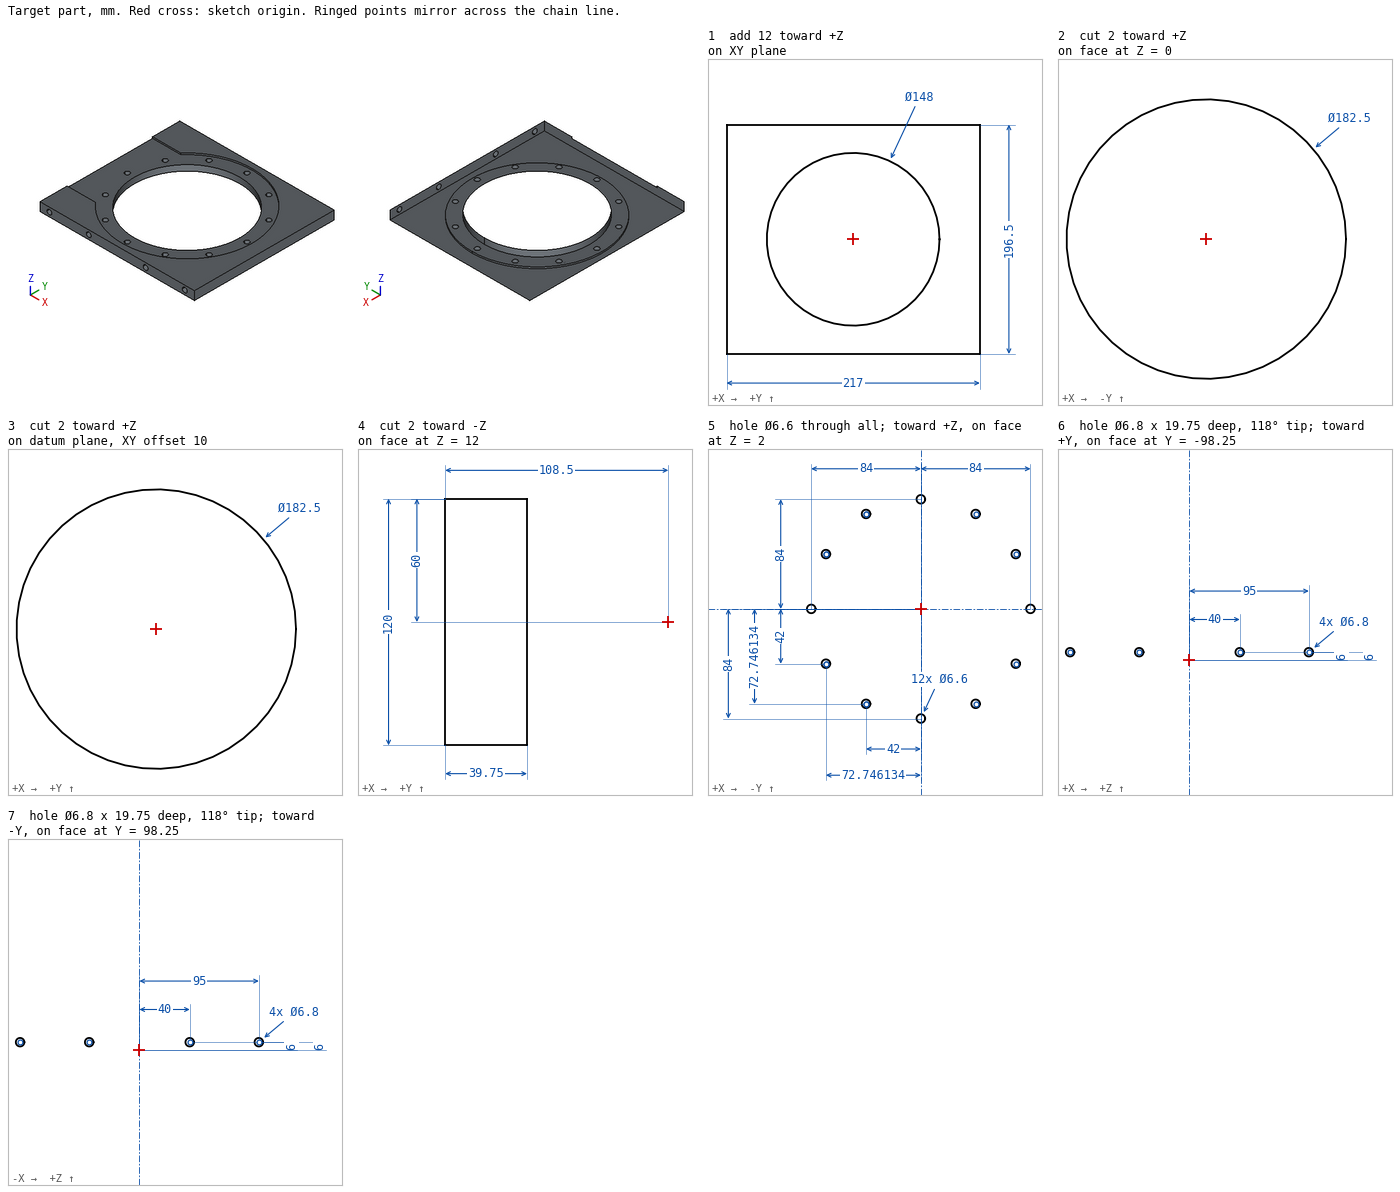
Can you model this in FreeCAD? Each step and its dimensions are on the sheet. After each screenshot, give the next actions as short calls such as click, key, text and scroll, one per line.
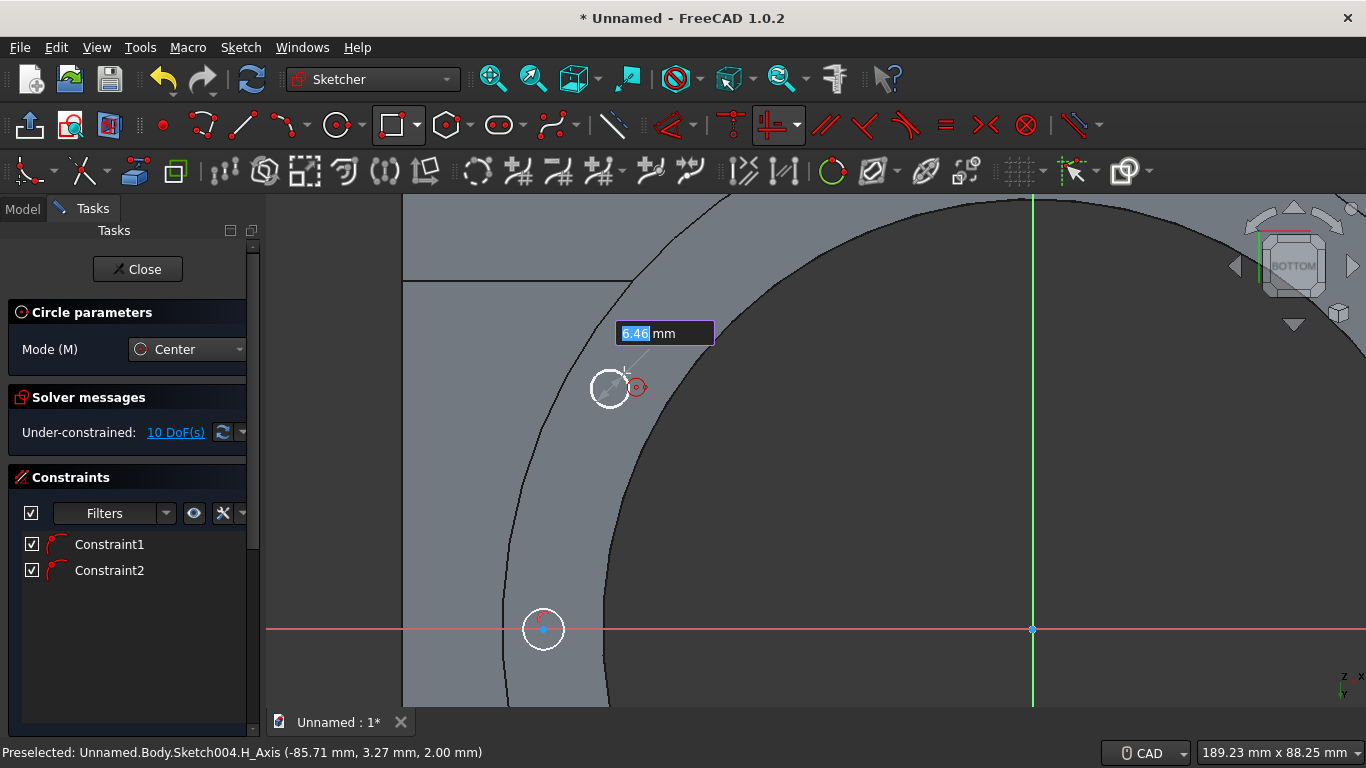
click(624, 372)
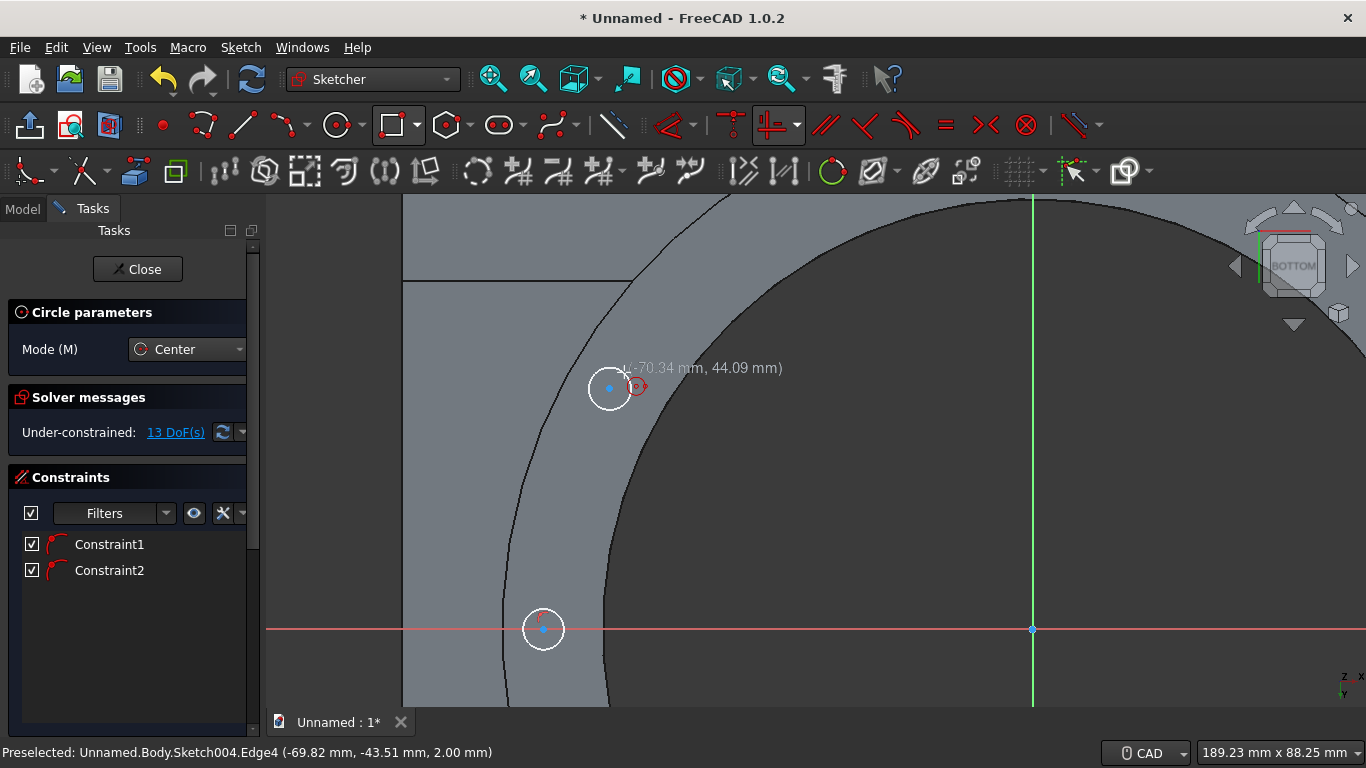
scroll(625, 373, down, 6)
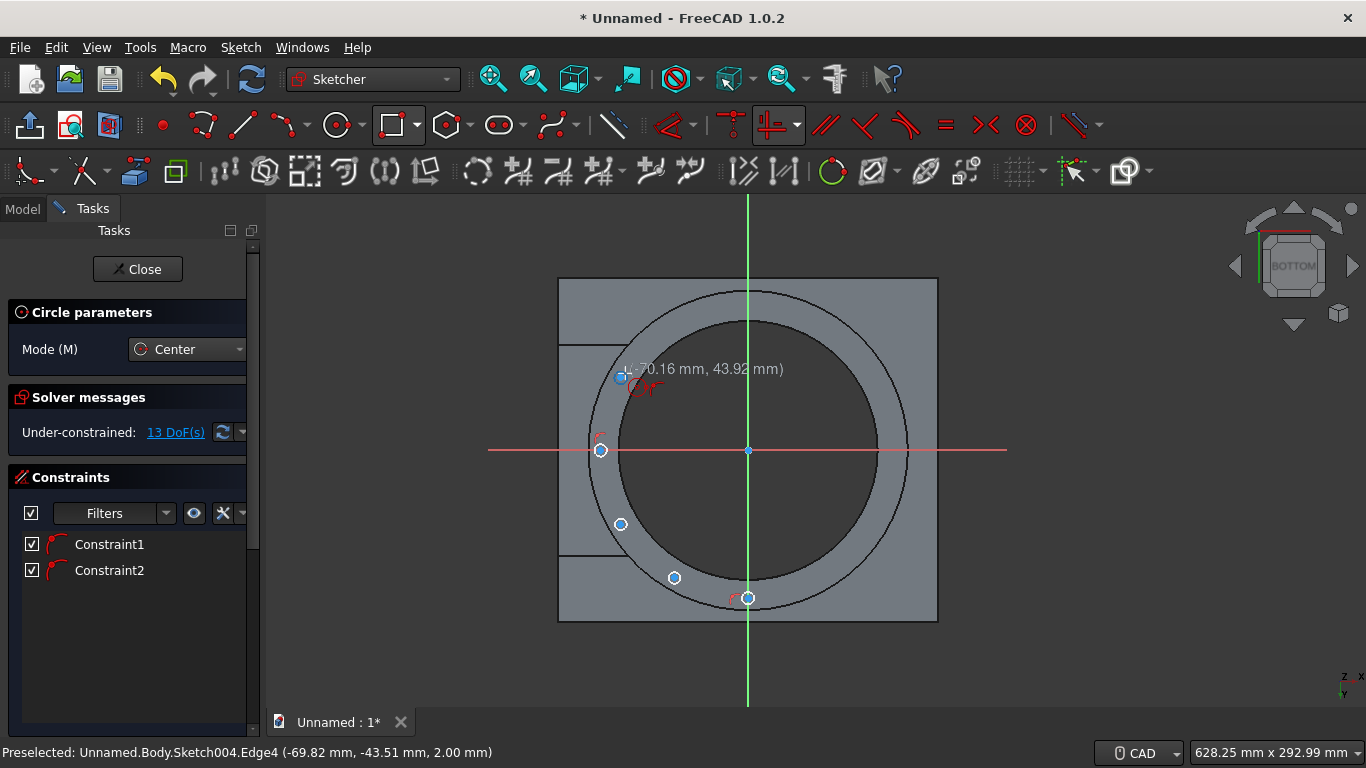
scroll(675, 323, up, 7)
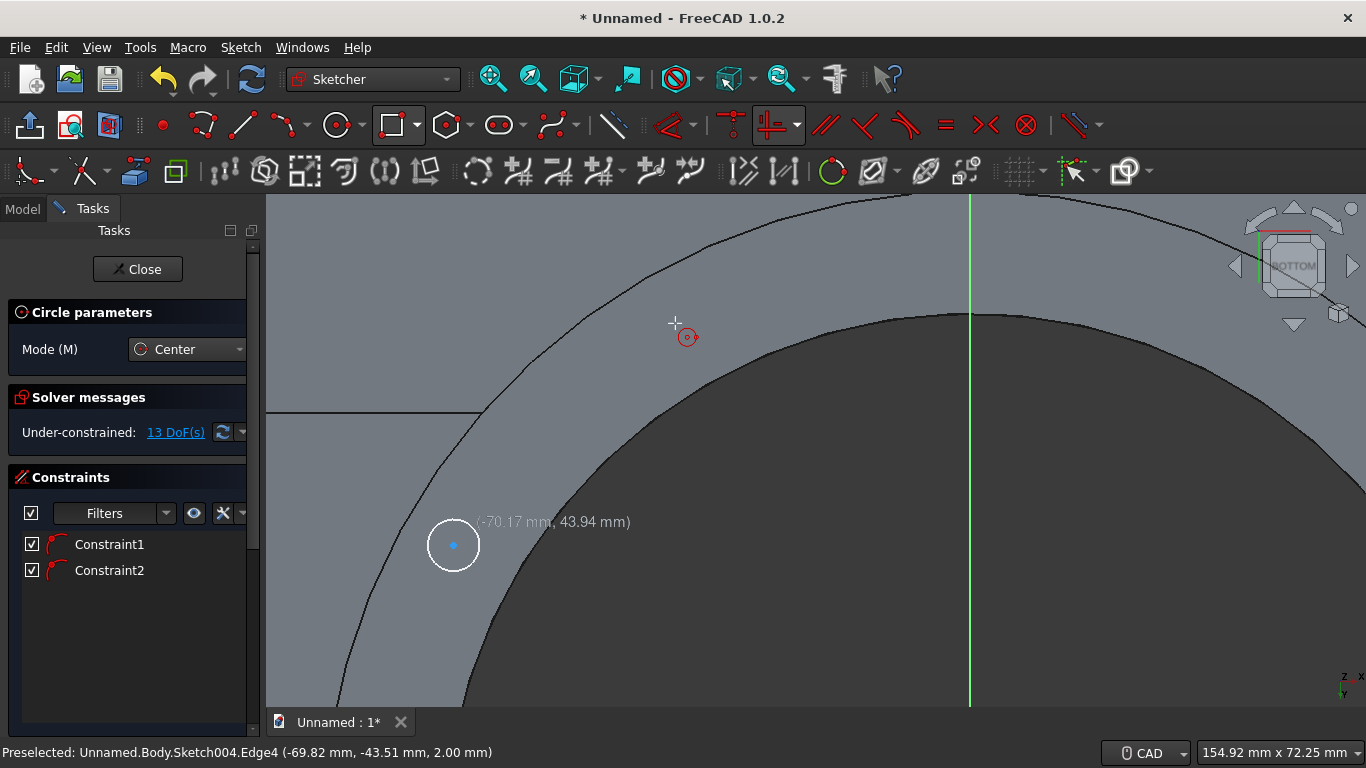
scroll(675, 323, down, 7)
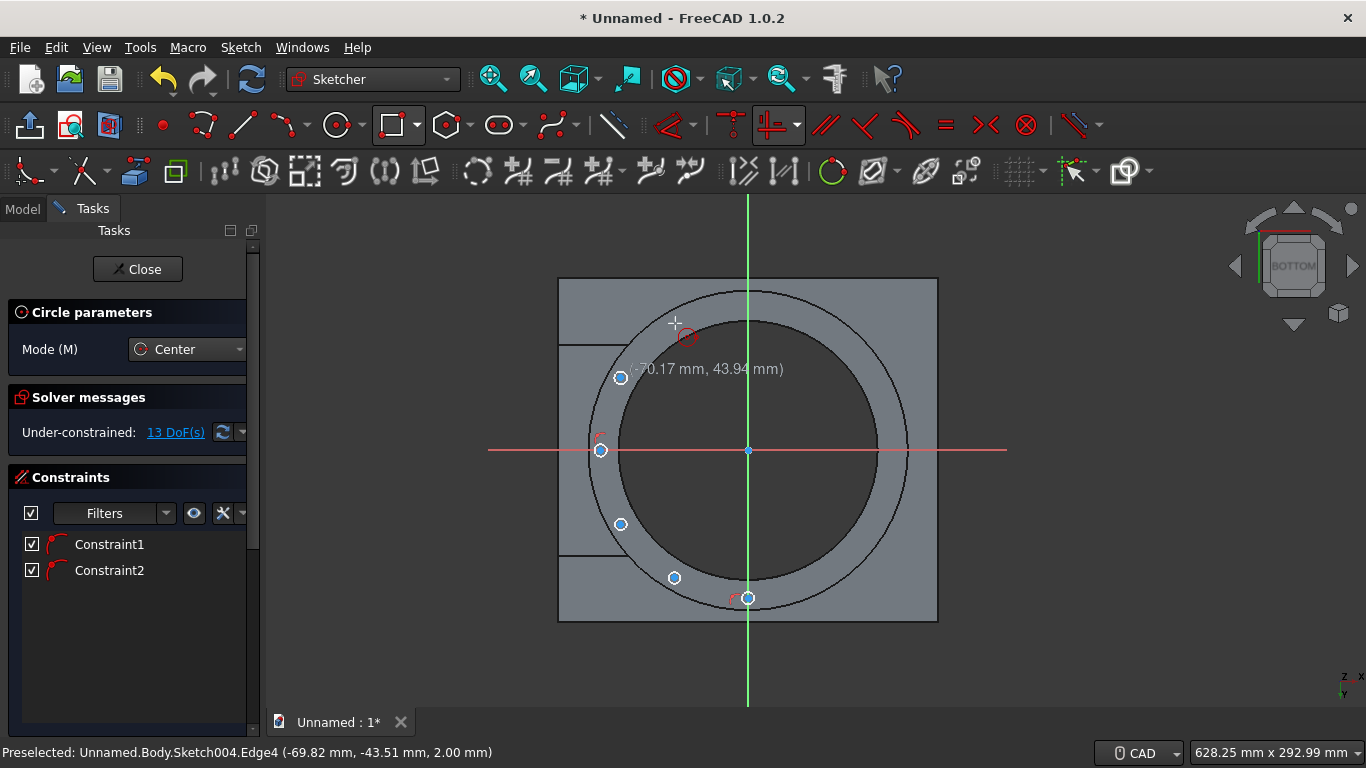
click(675, 323)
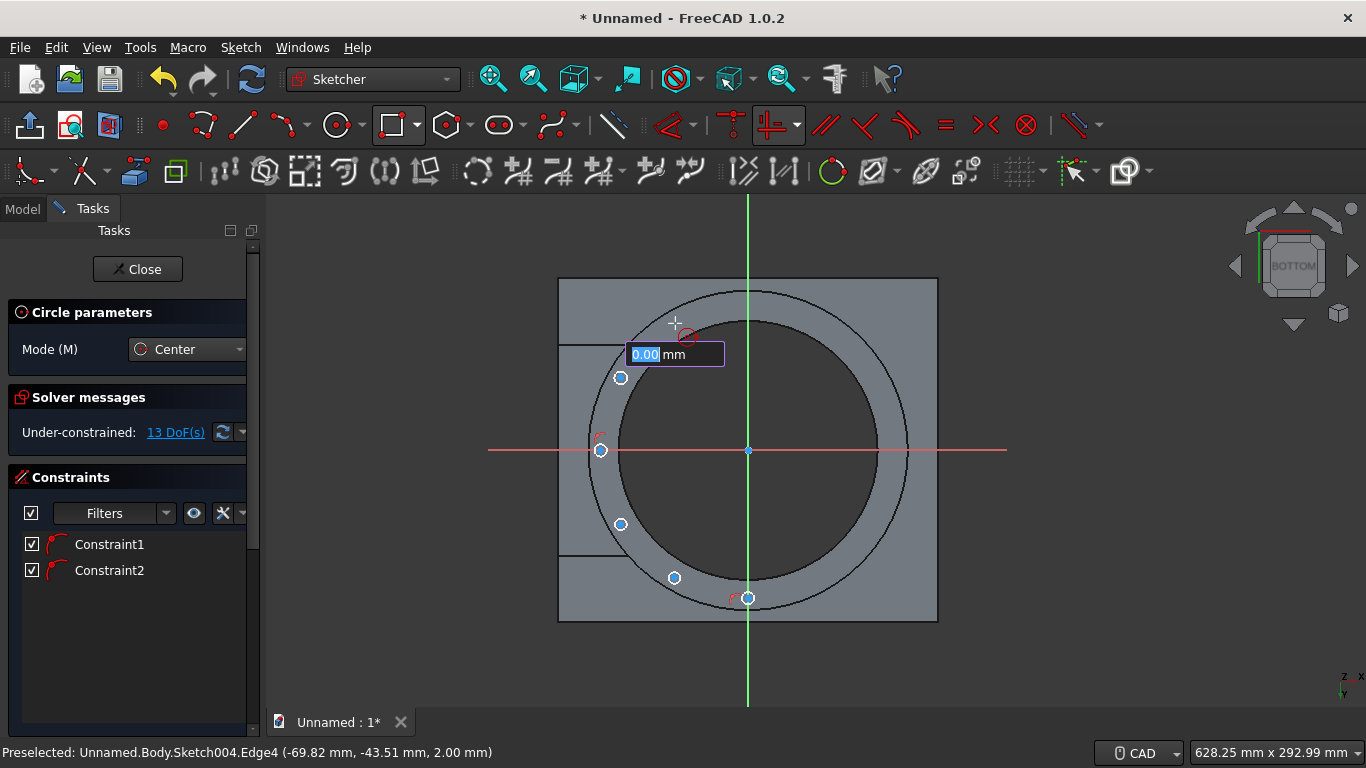
scroll(679, 319, up, 6)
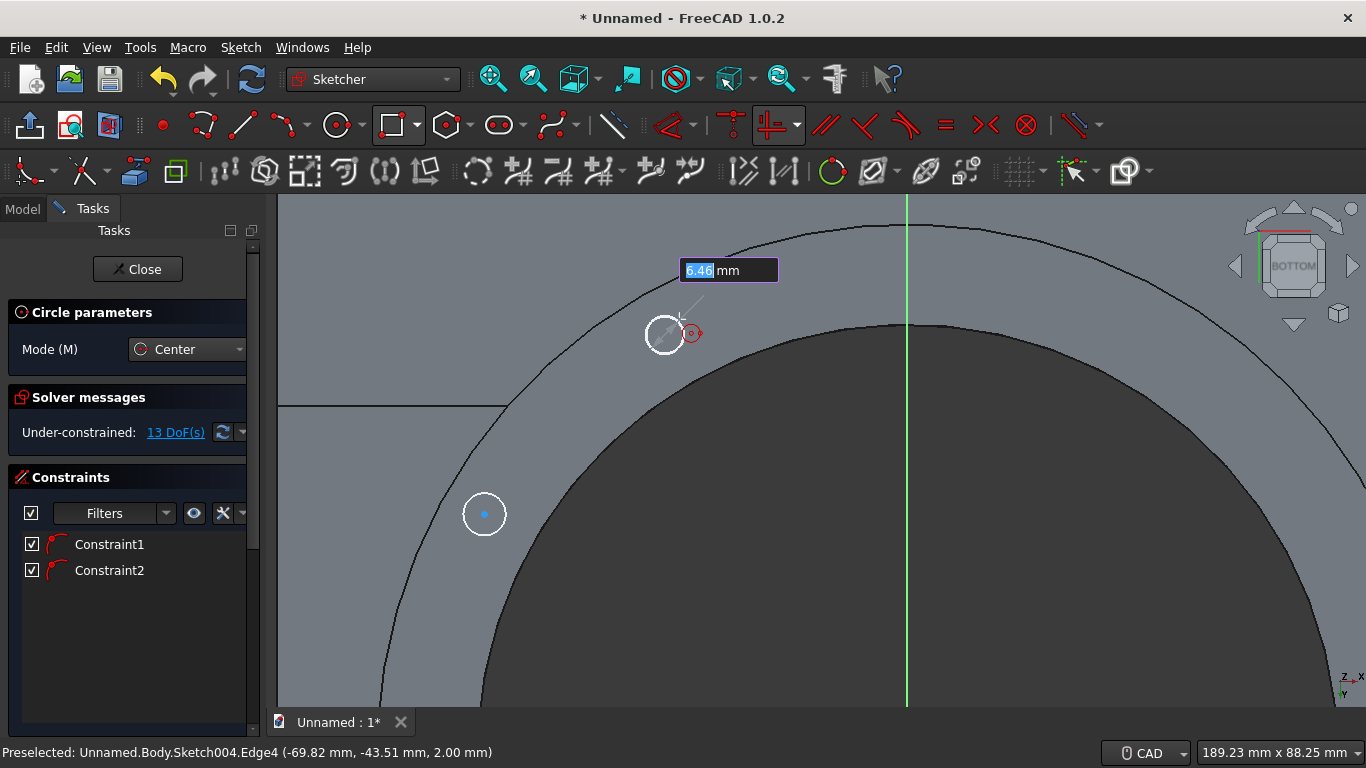
click(677, 318)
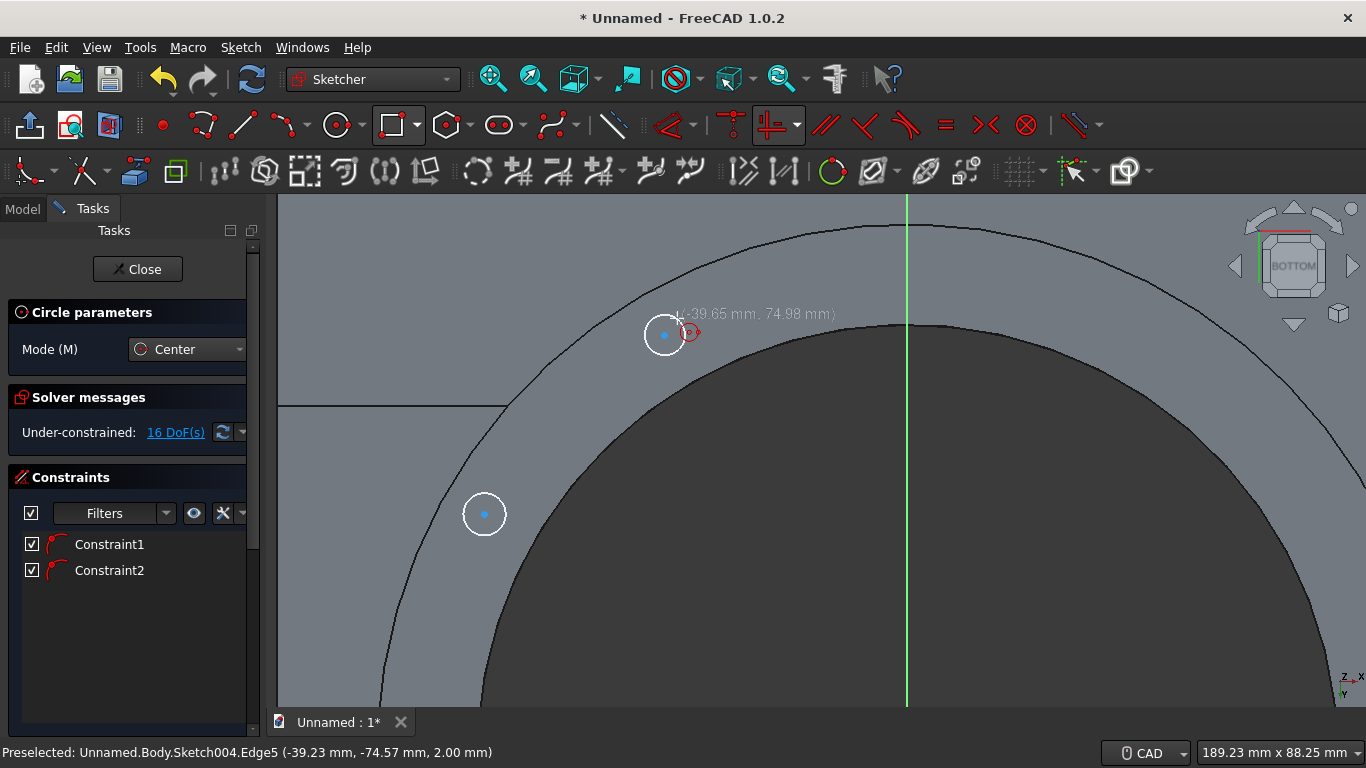
click(907, 267)
click(925, 260)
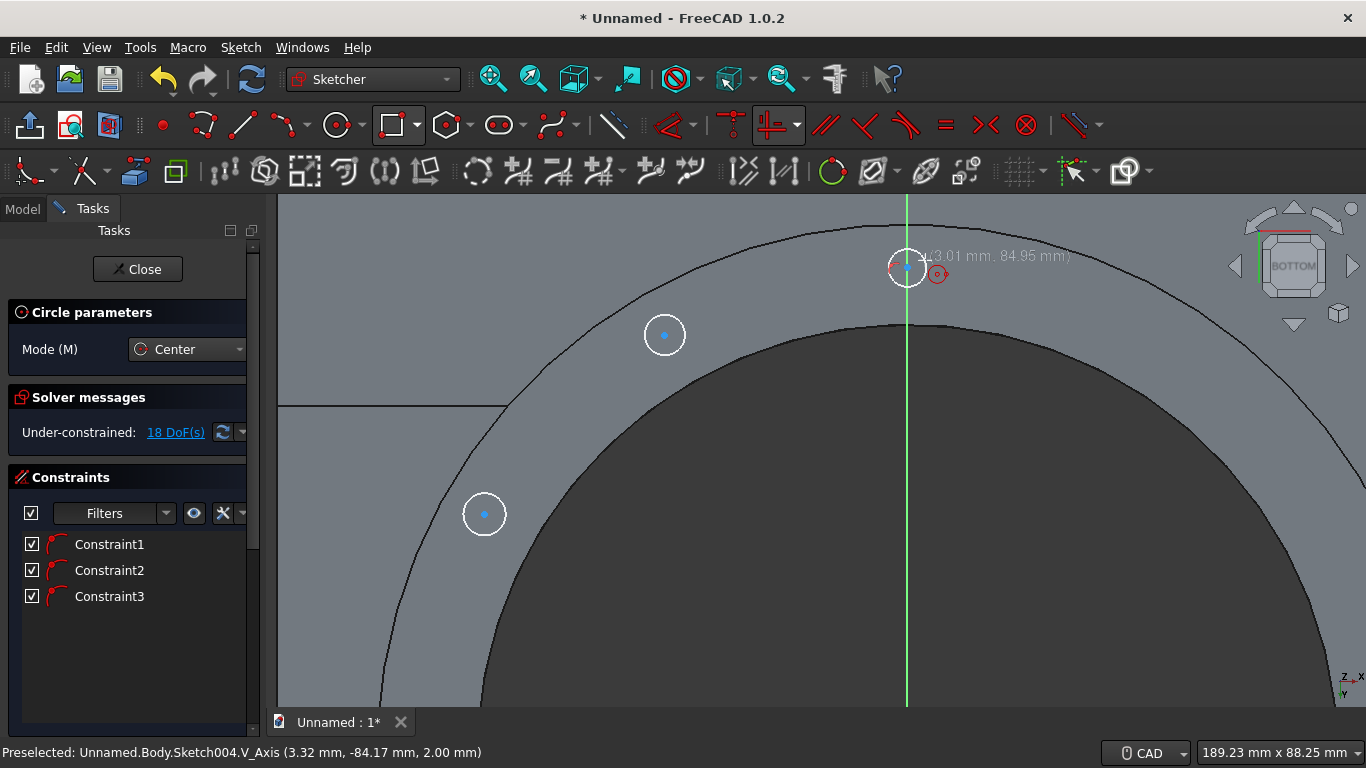
click(1152, 332)
click(1165, 318)